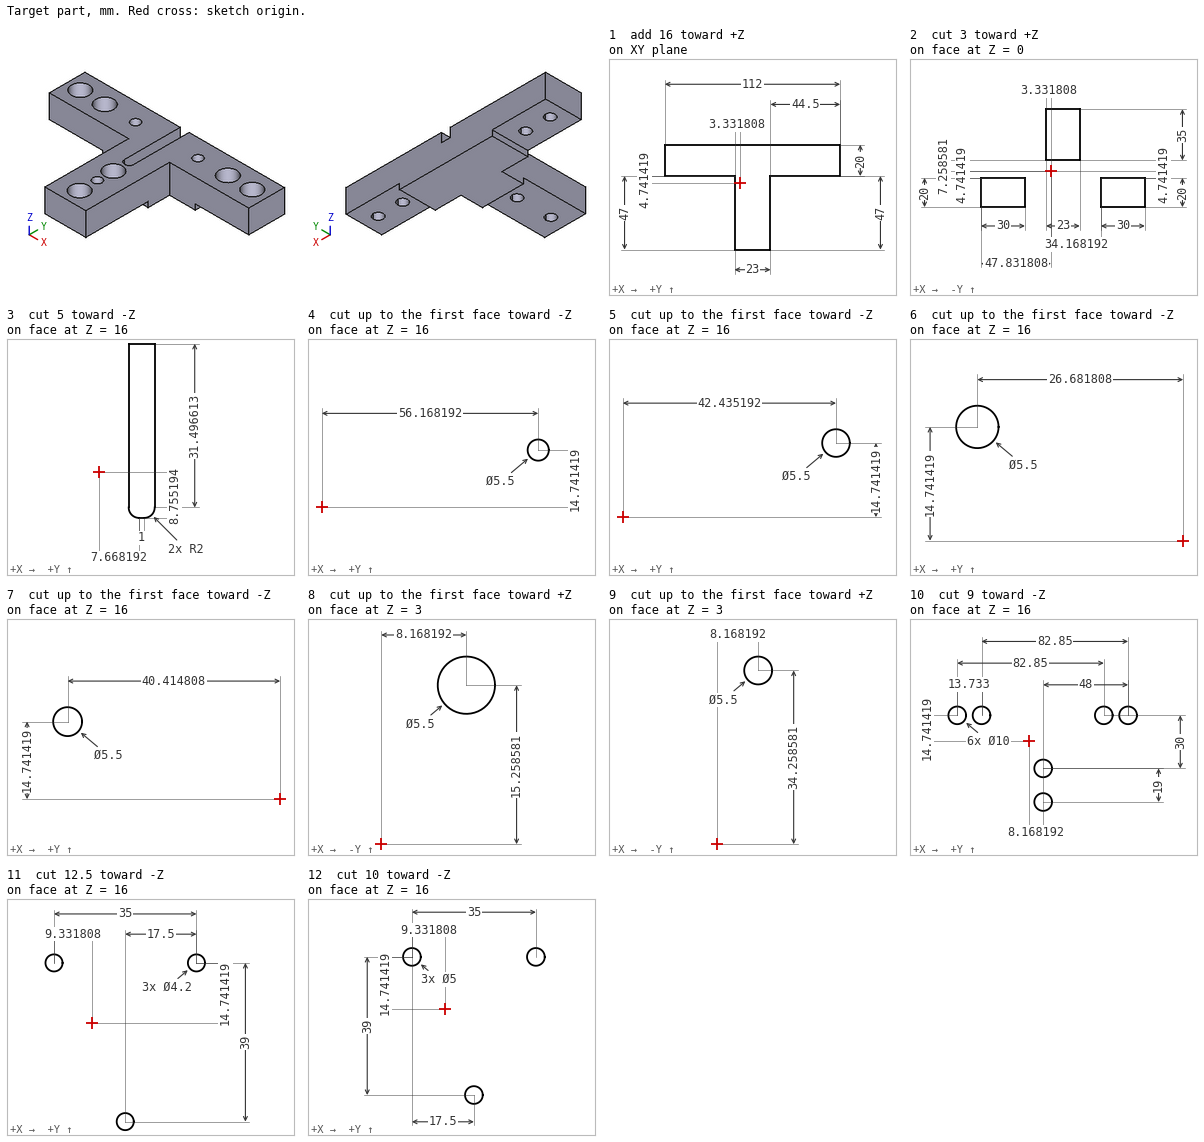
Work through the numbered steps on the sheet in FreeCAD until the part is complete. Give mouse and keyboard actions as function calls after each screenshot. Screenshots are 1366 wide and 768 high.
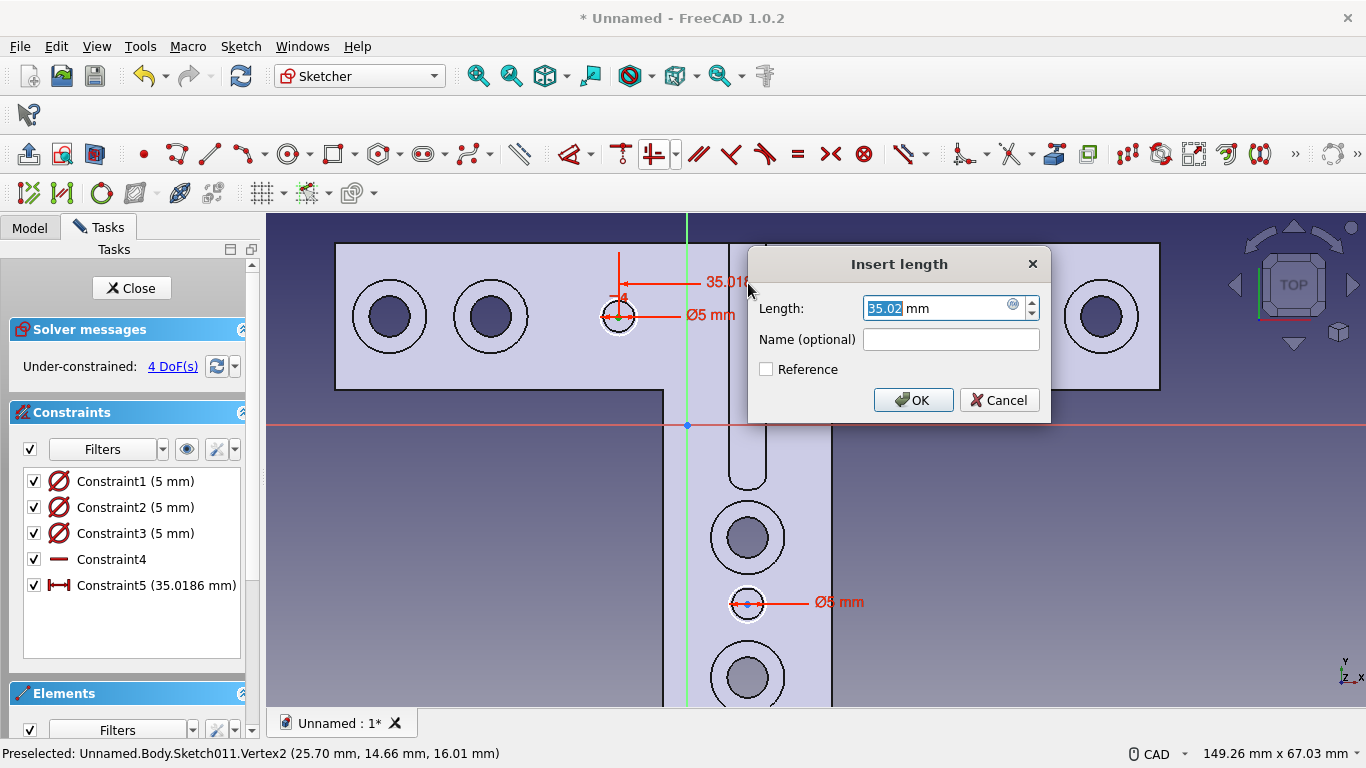
text(35)
key(Return)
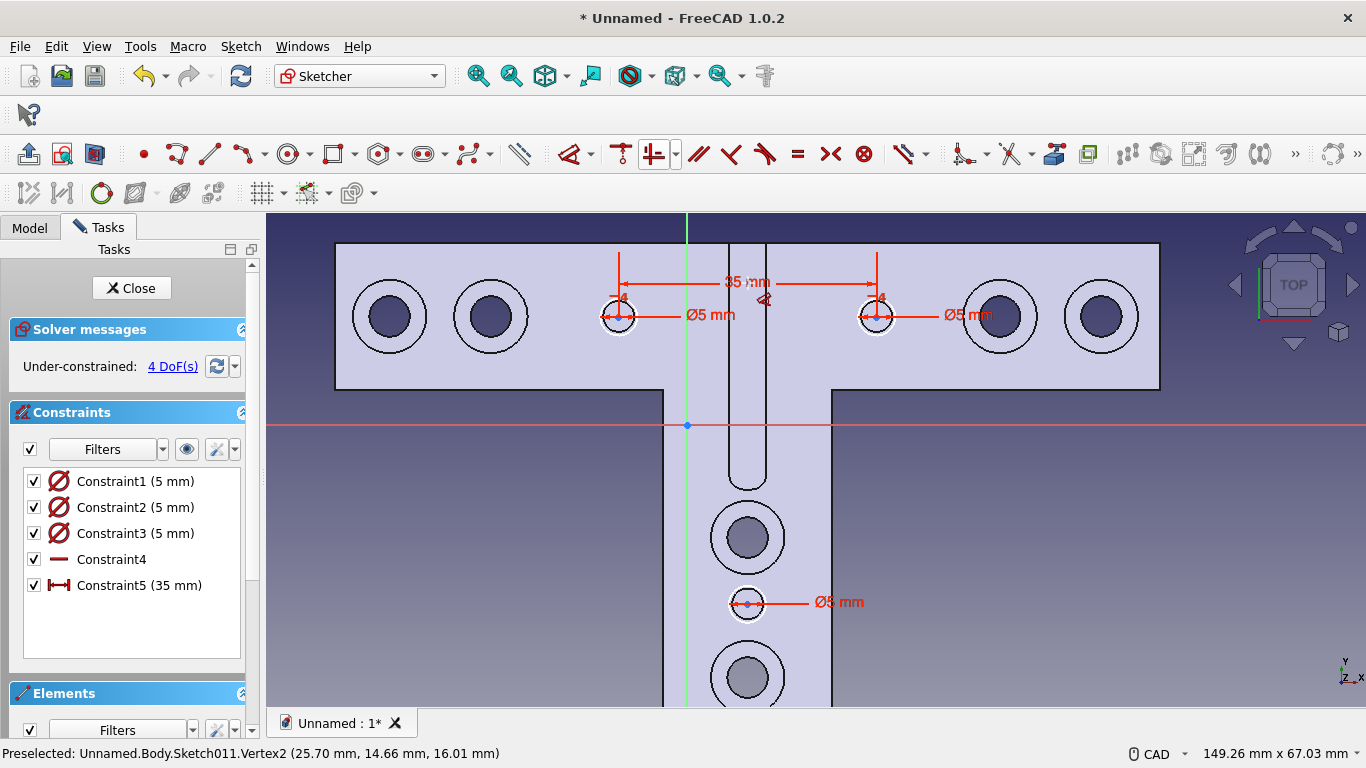
click(619, 317)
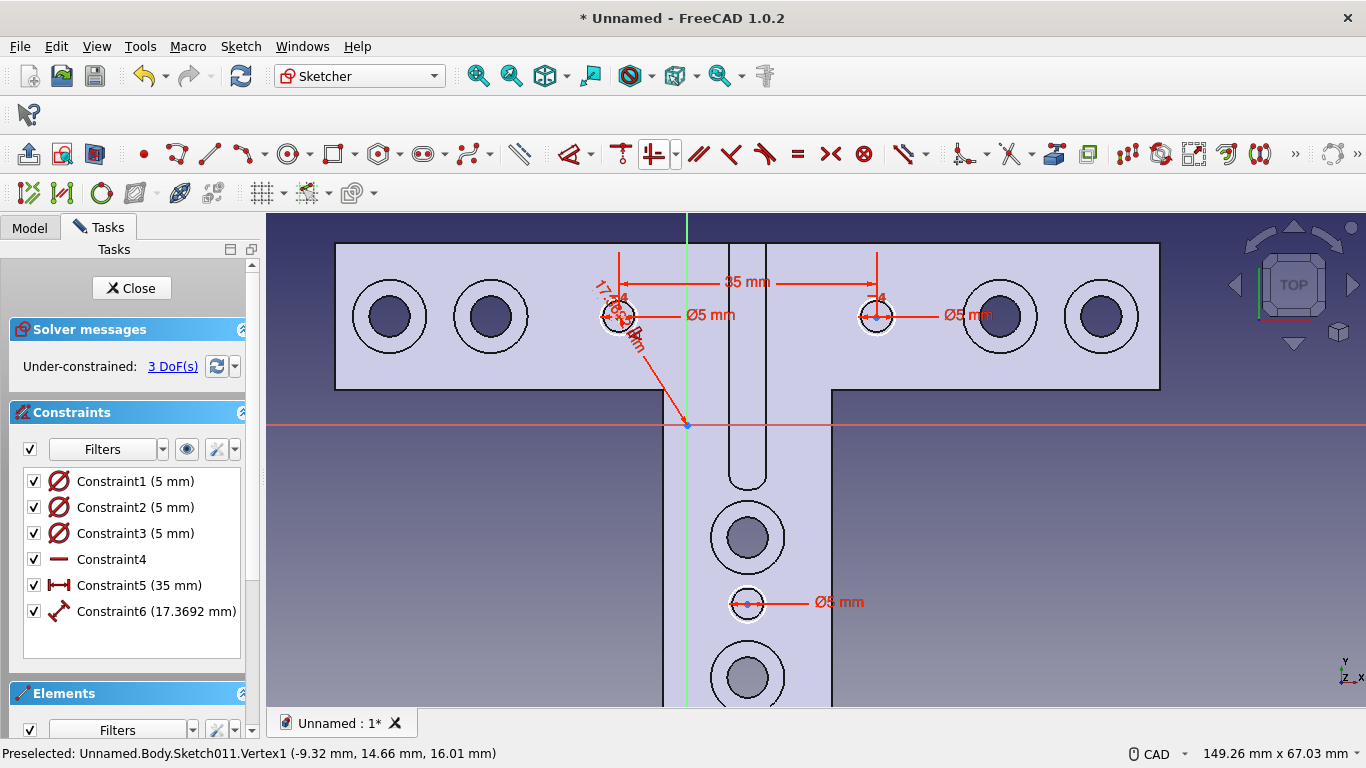
click(747, 604)
click(585, 461)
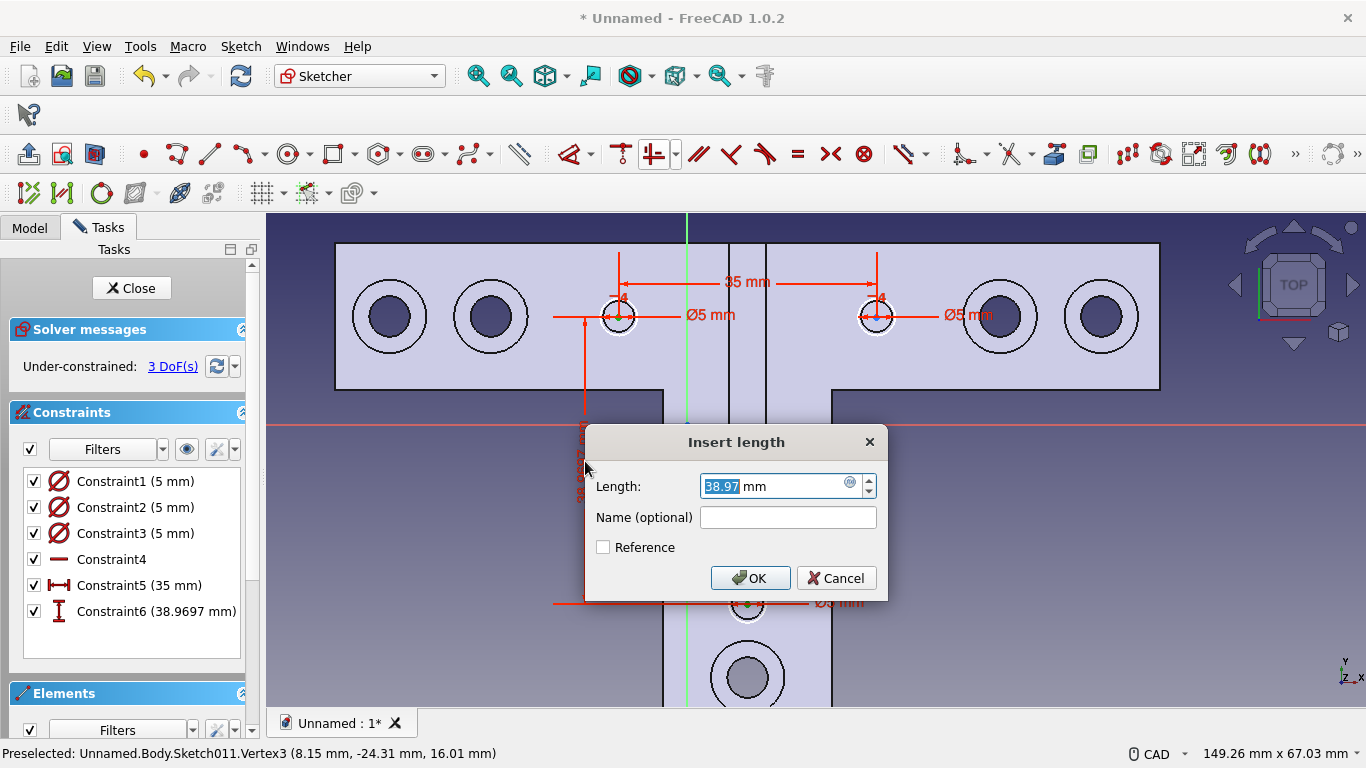
text(39)
key(Return)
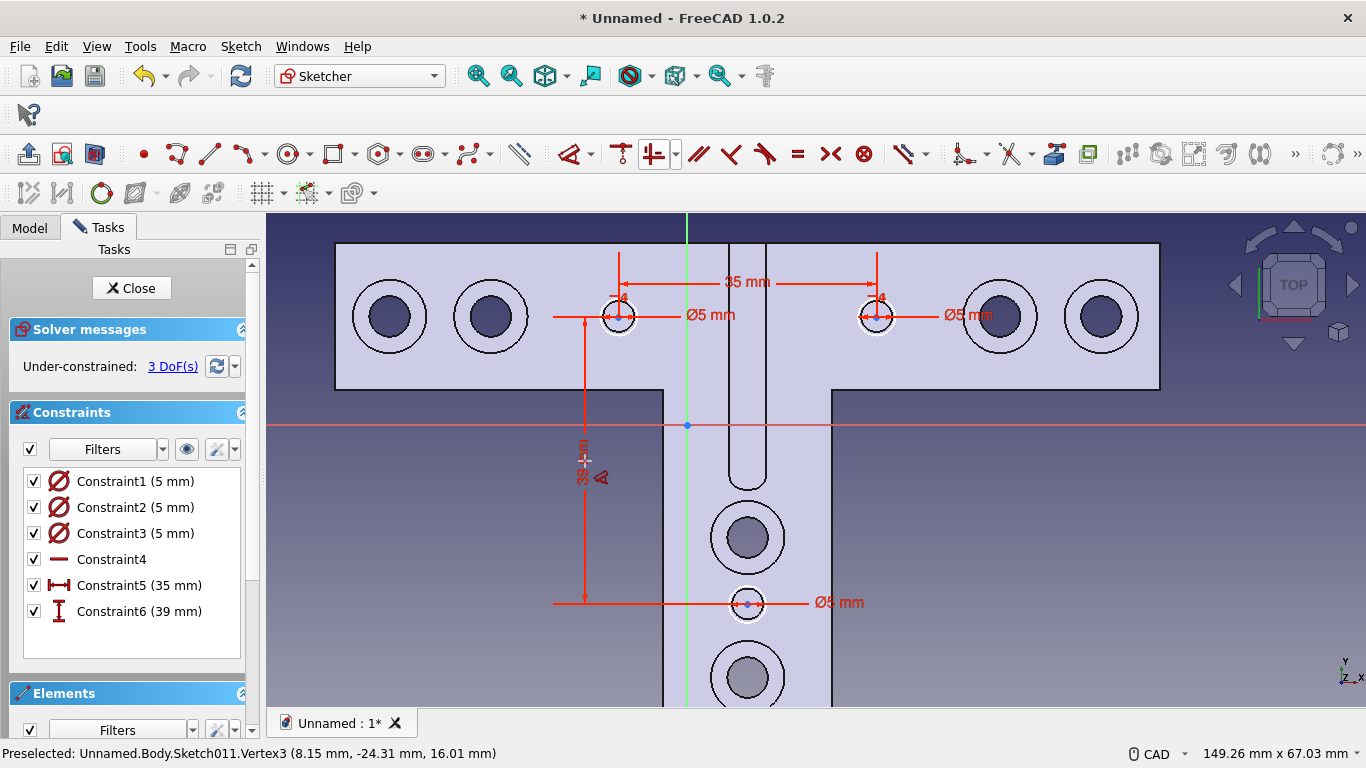
click(619, 317)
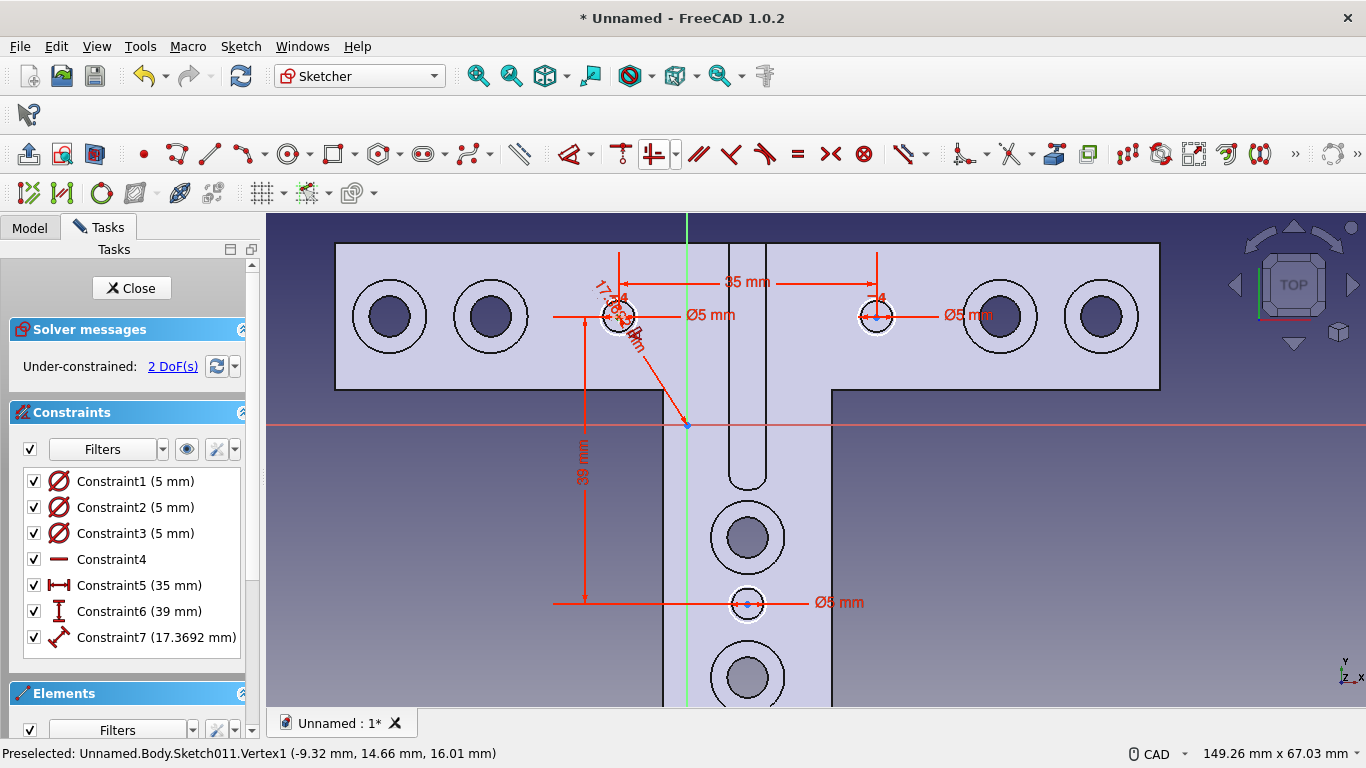
click(747, 604)
click(654, 638)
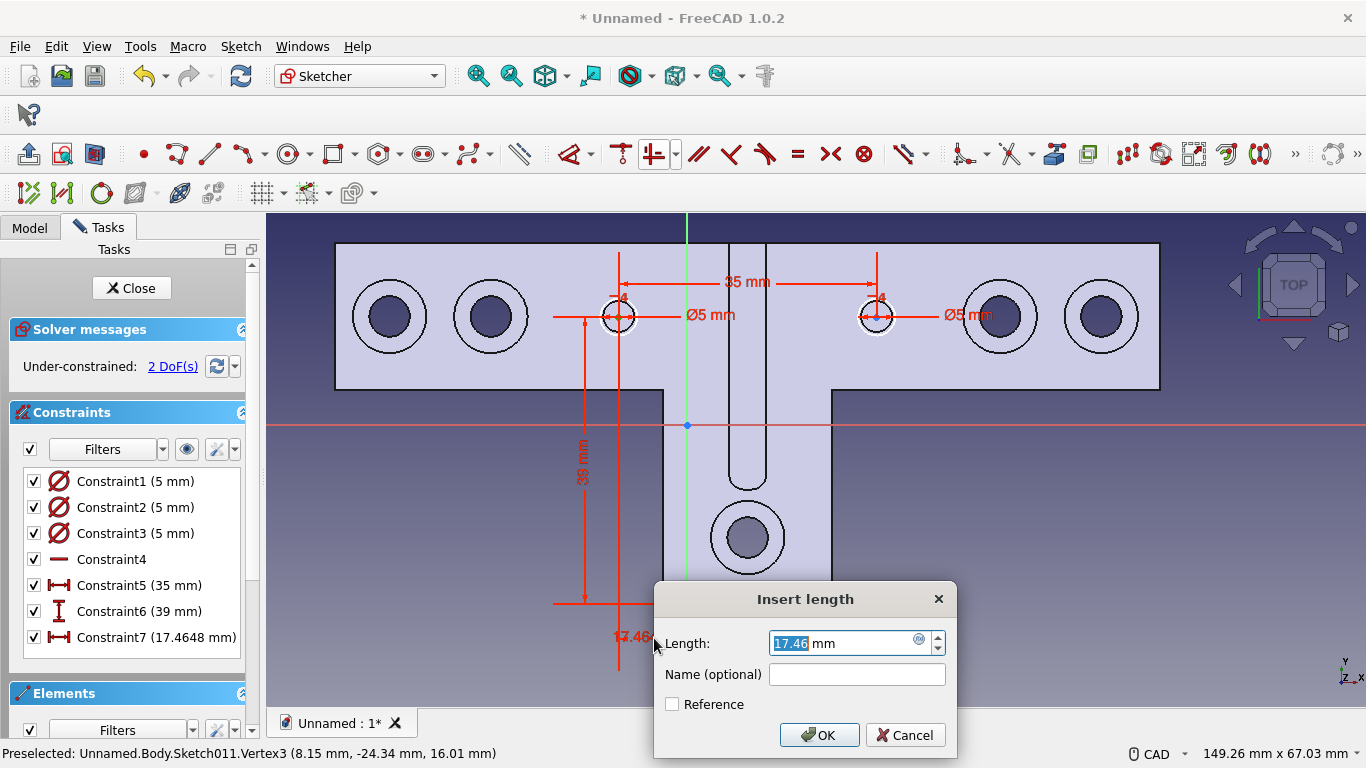
text(17.5)
key(Return)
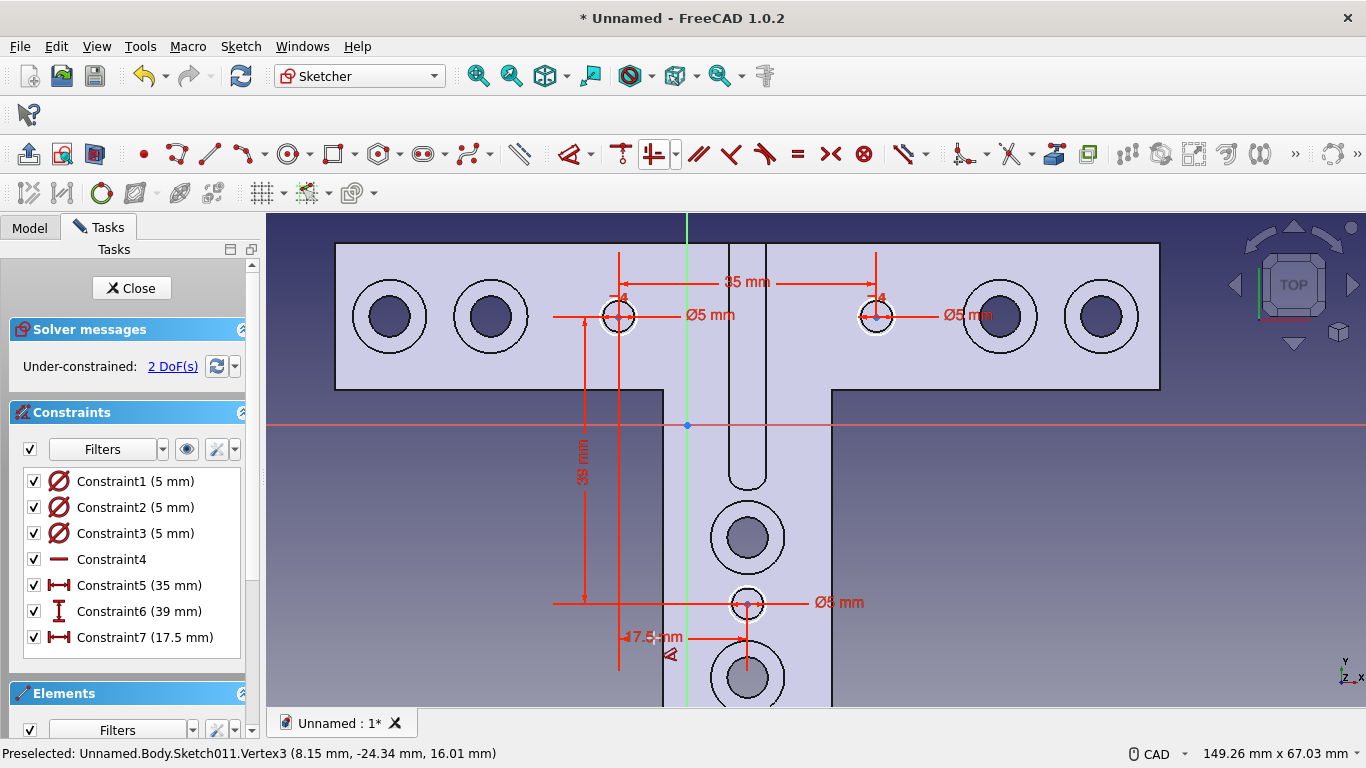
click(619, 317)
click(653, 283)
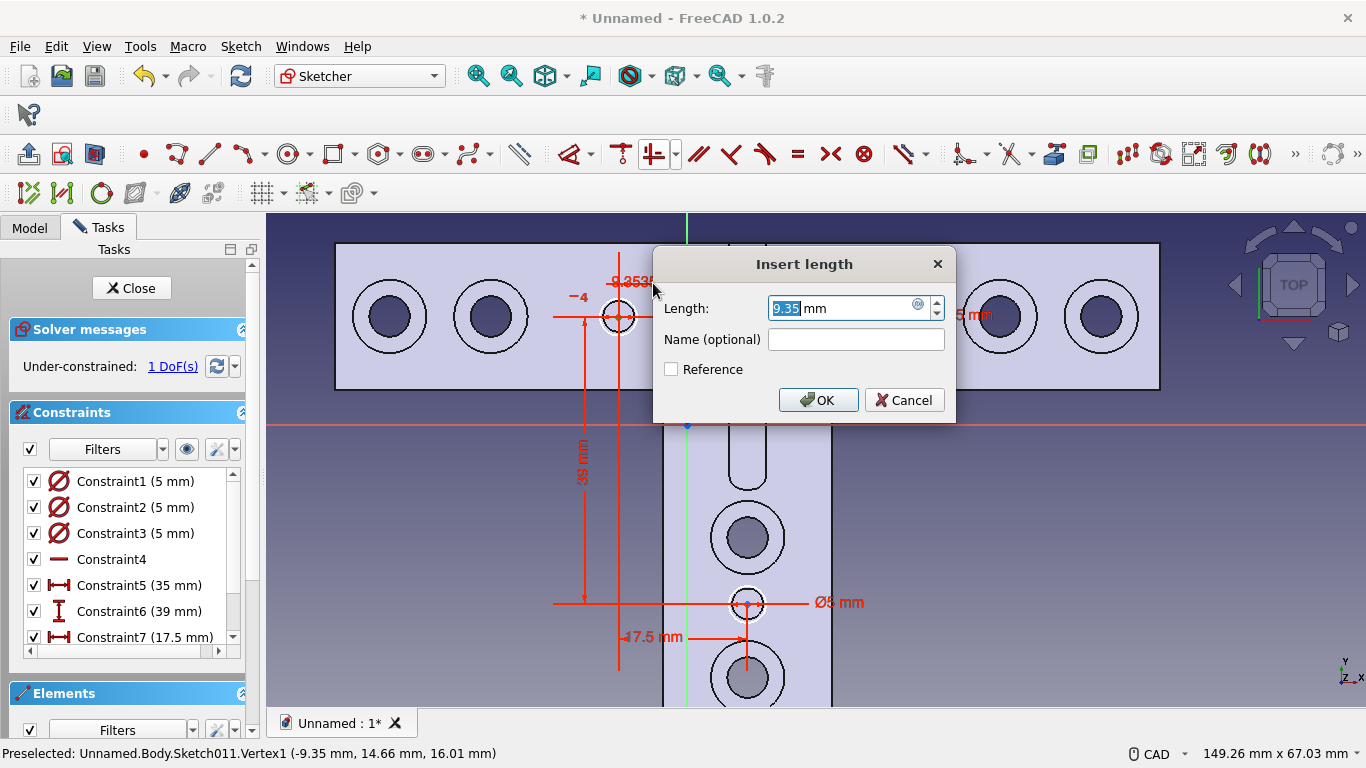
text(9.331808)
key(Return)